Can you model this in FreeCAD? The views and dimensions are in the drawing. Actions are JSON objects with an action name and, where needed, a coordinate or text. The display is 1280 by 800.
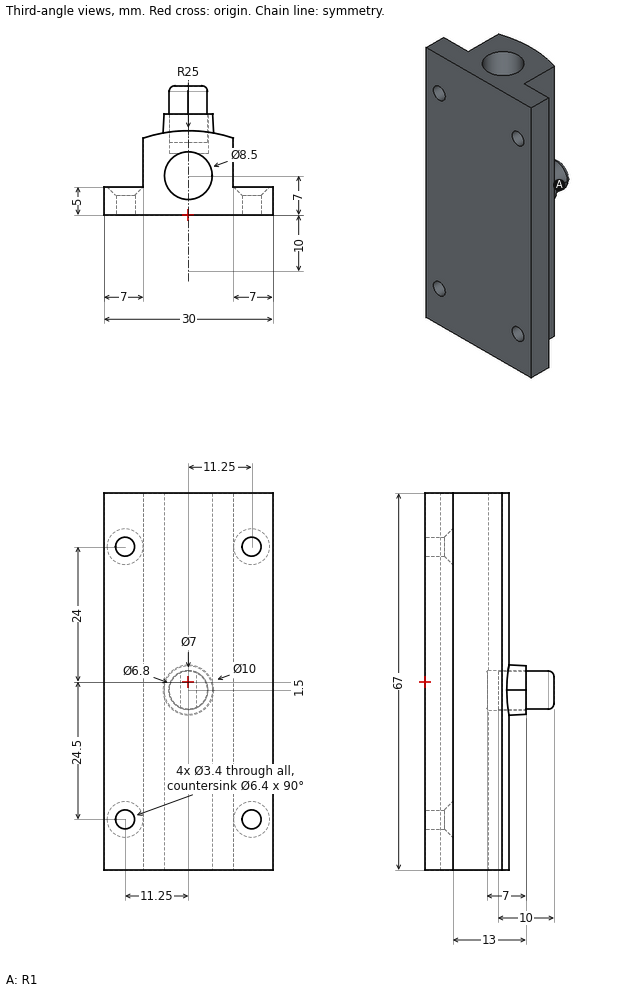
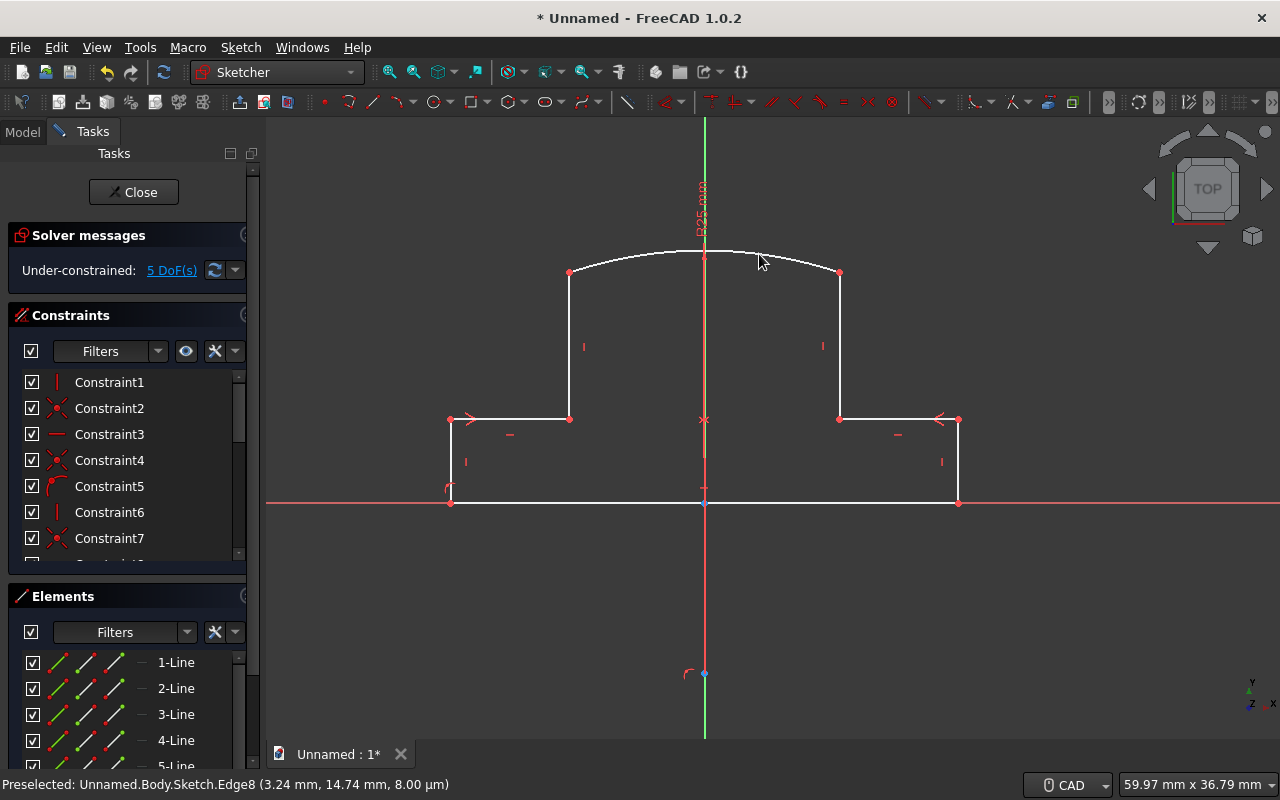
{"action": "left_click", "coordinate": [534, 419]}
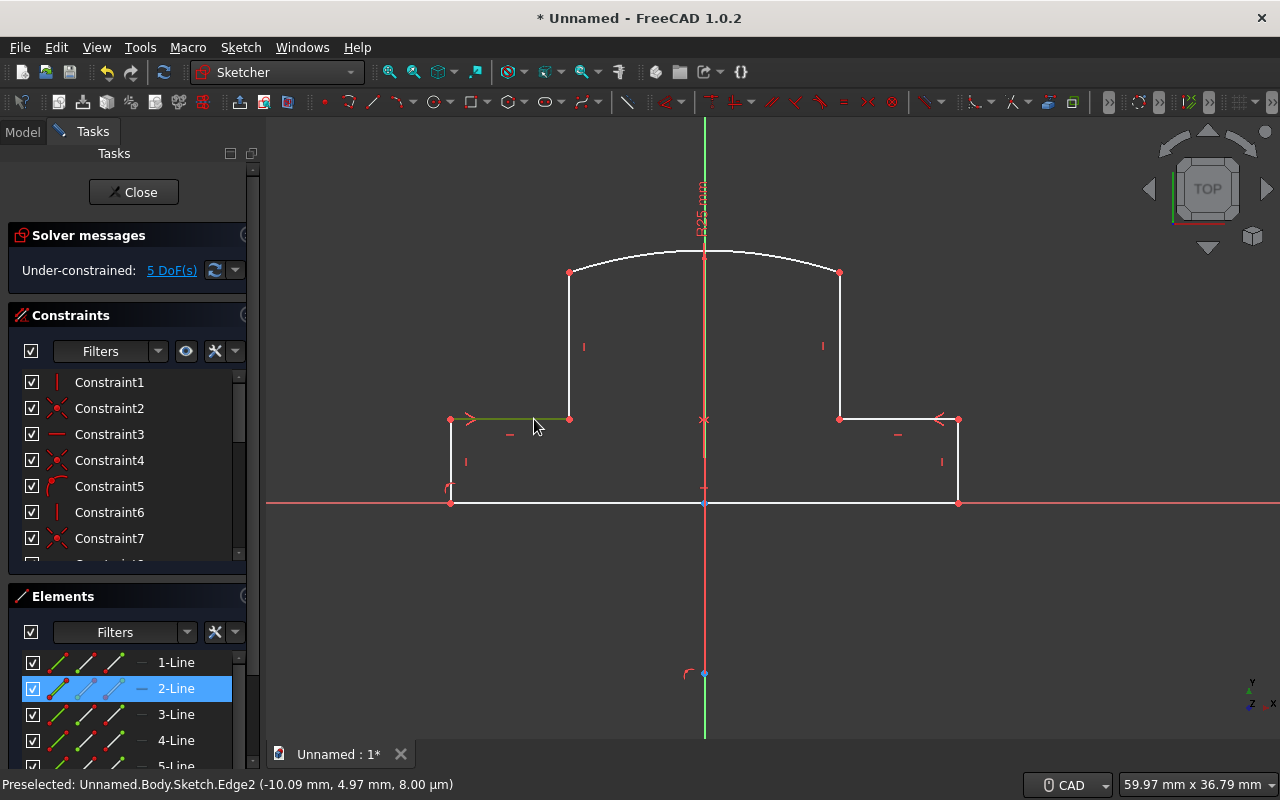
{"action": "left_click", "coordinate": [684, 102]}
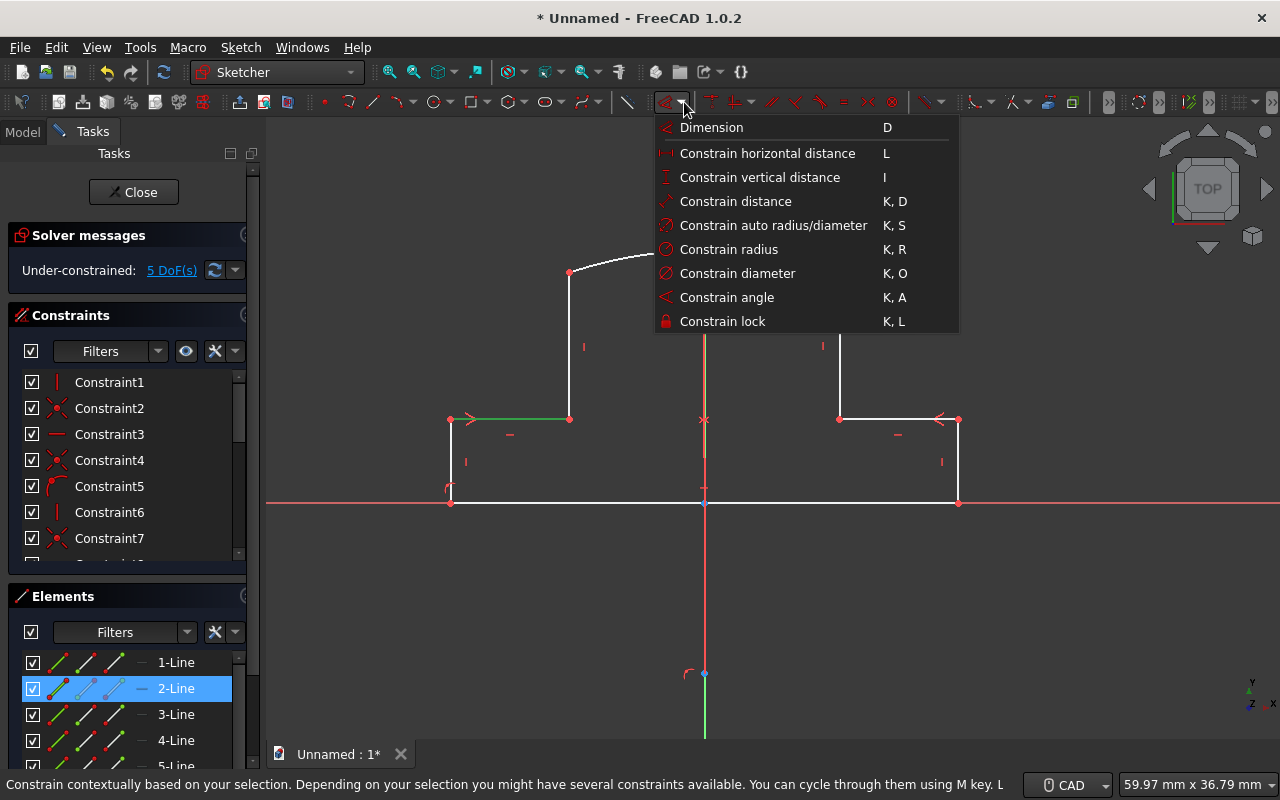
{"action": "left_click", "coordinate": [807, 153]}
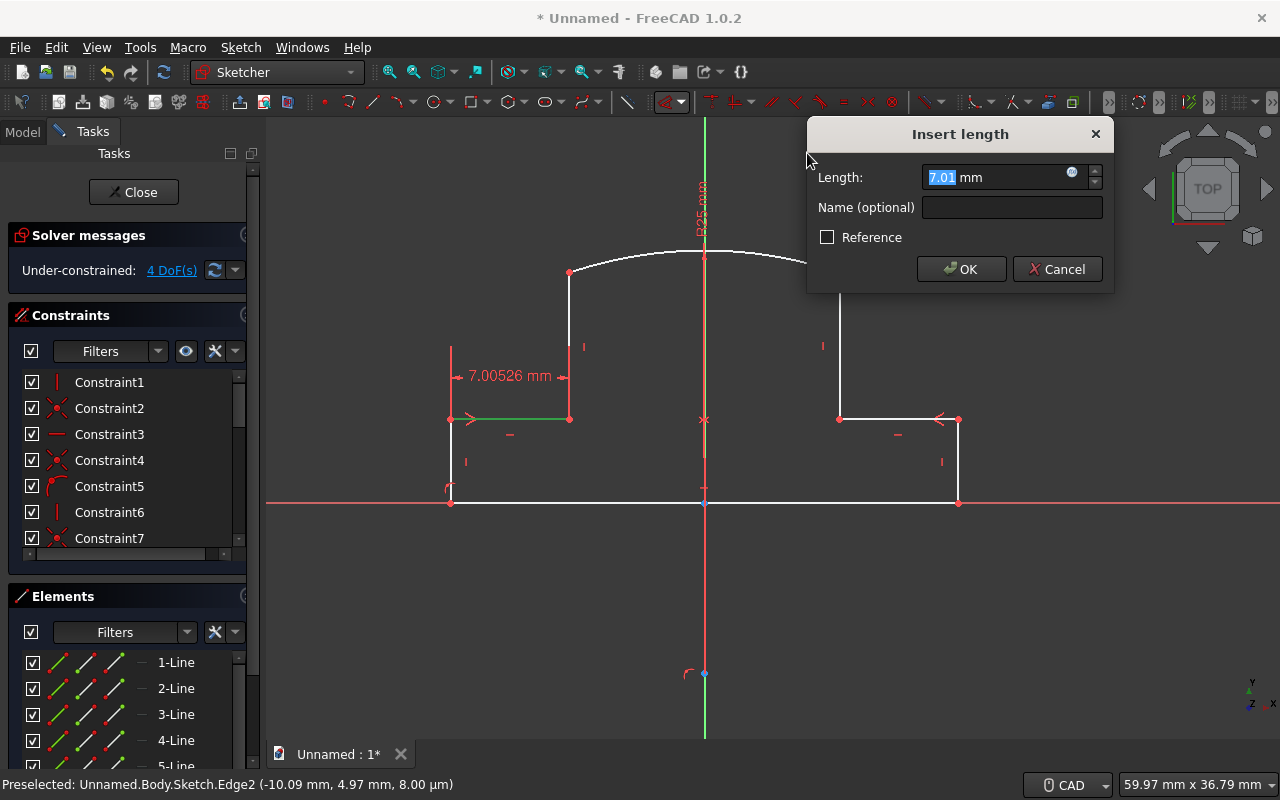
{"action": "type", "text": "7"}
{"action": "key", "text": "Return"}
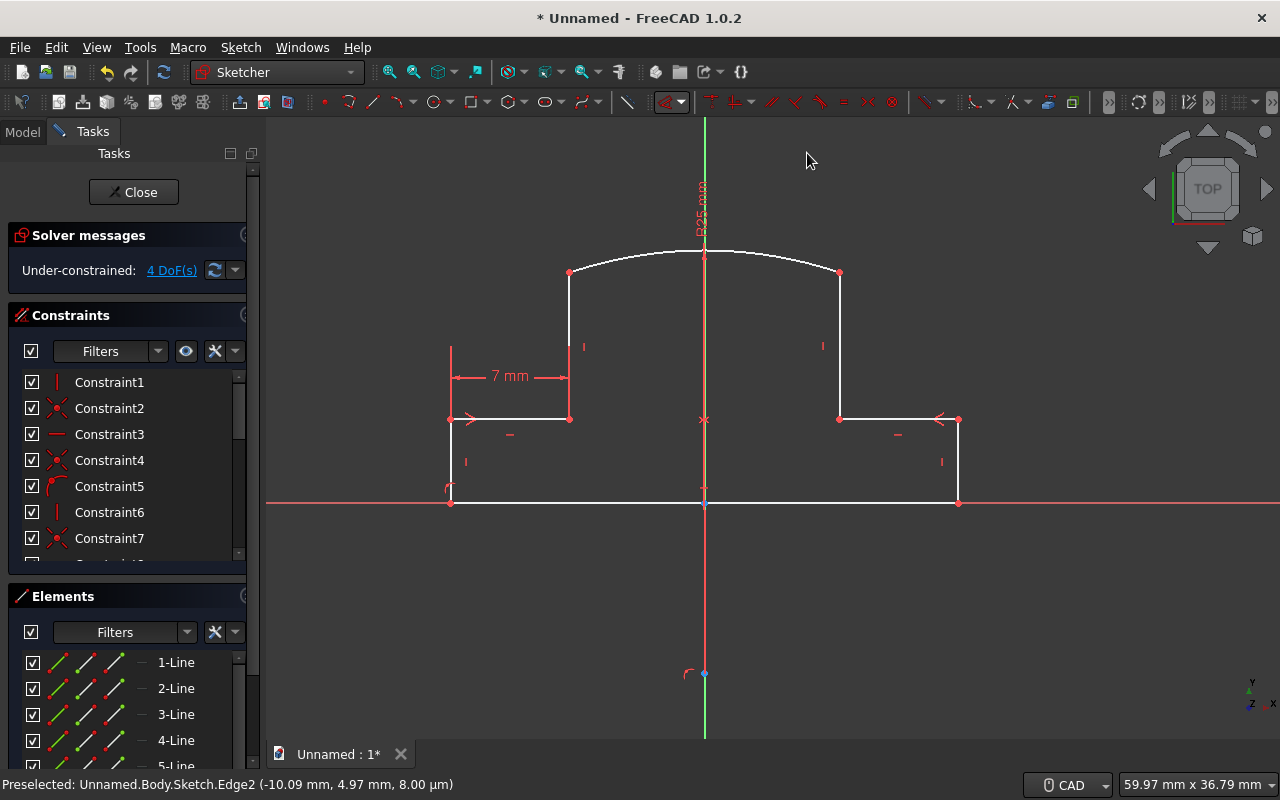
{"action": "left_click", "coordinate": [451, 444]}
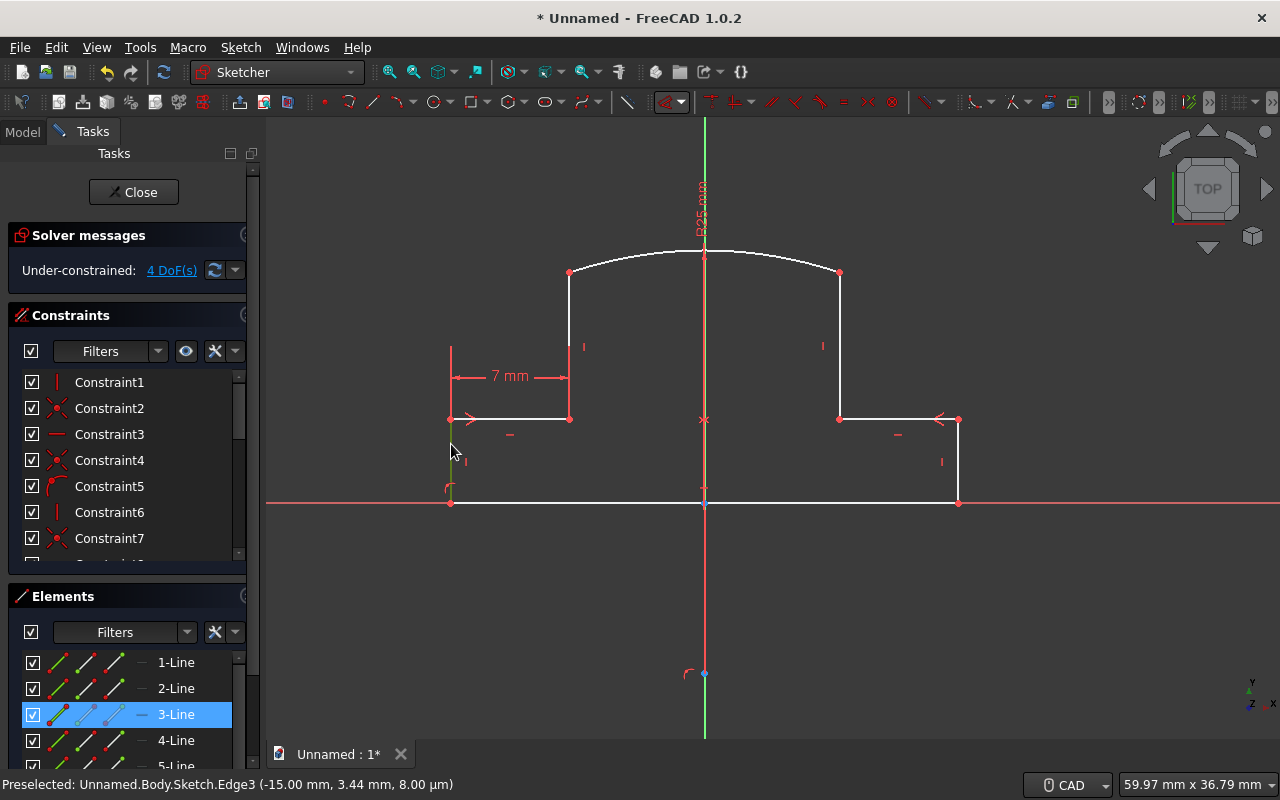
{"action": "key", "text": "i"}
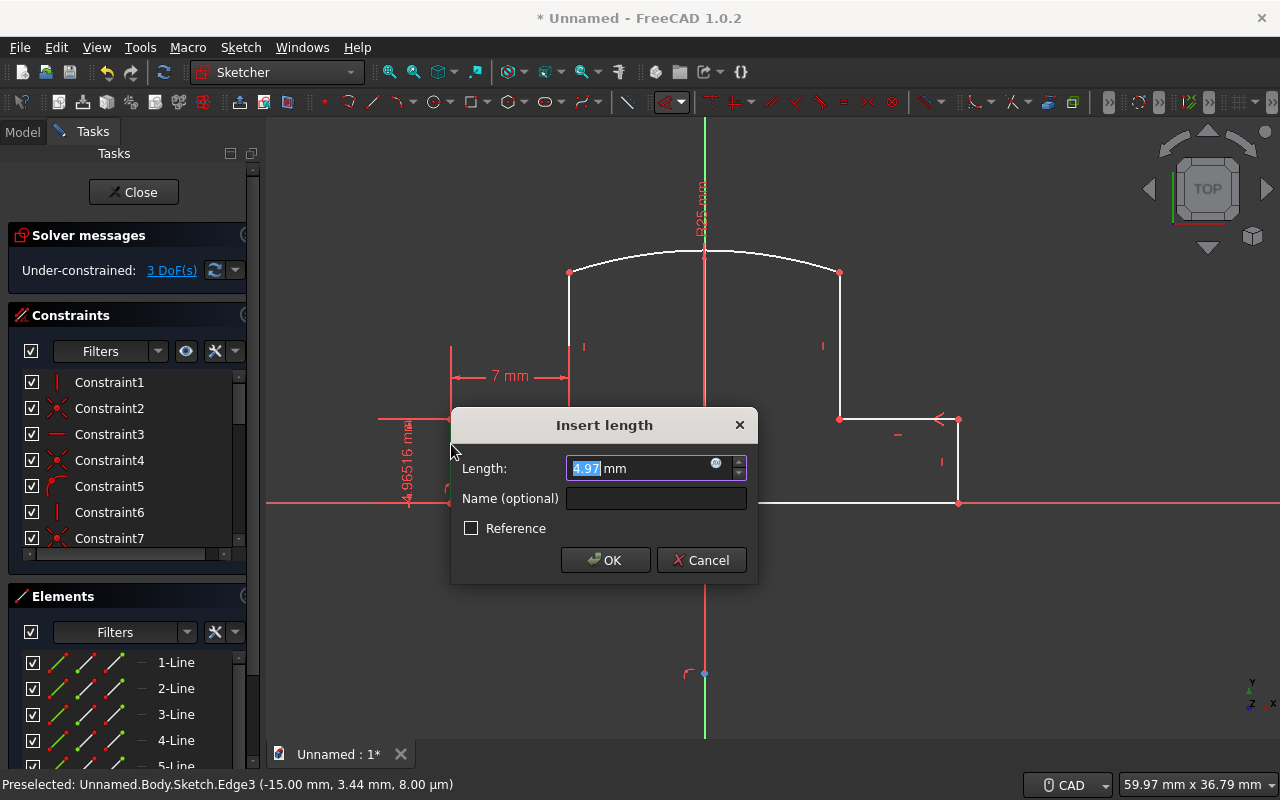
{"action": "type", "text": "5"}
{"action": "key", "text": "Return"}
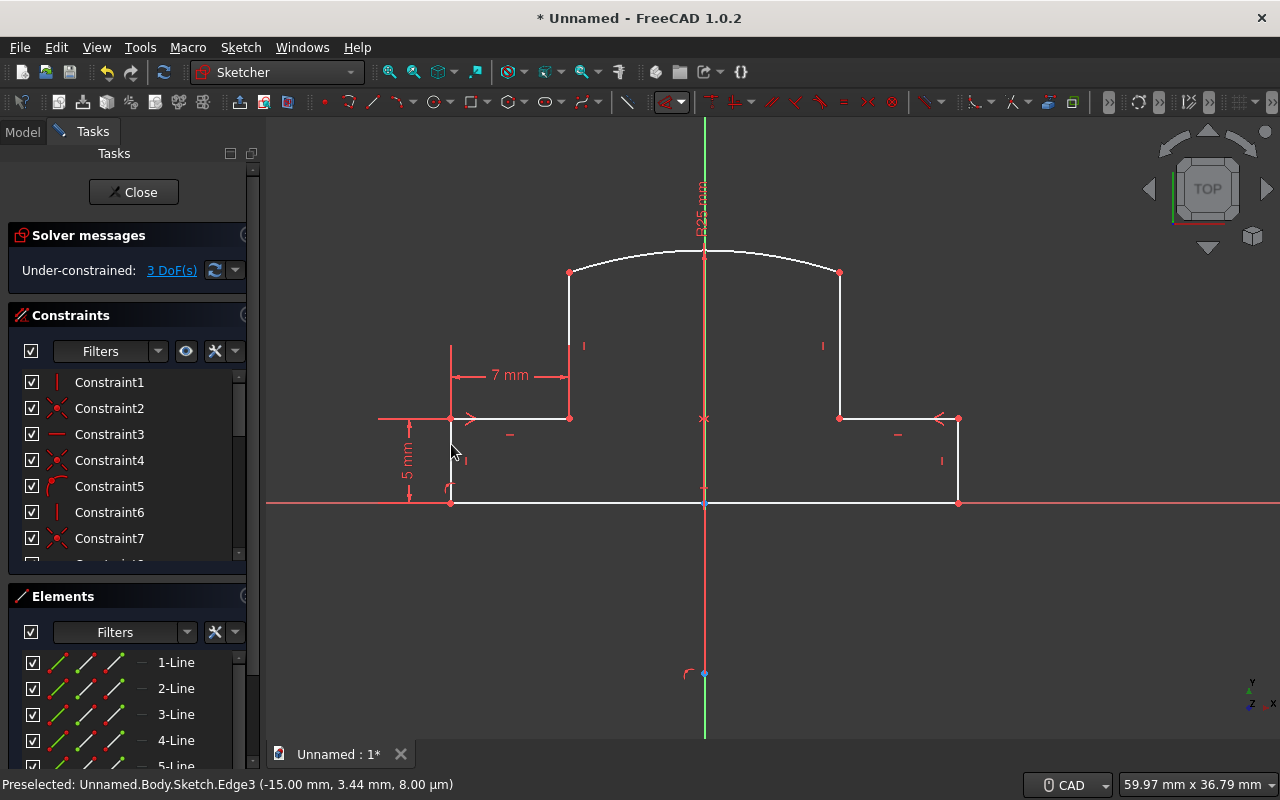
{"action": "left_click", "coordinate": [923, 419]}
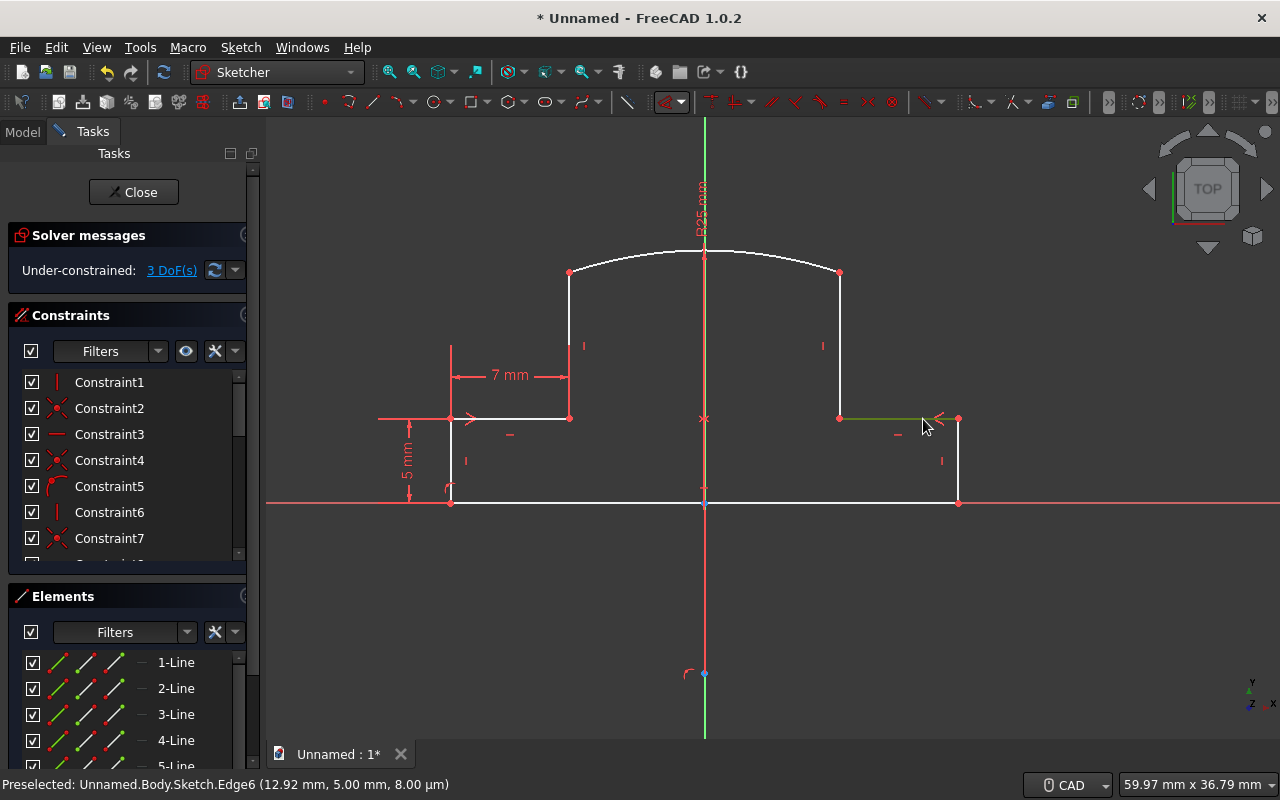
{"action": "key", "text": "l"}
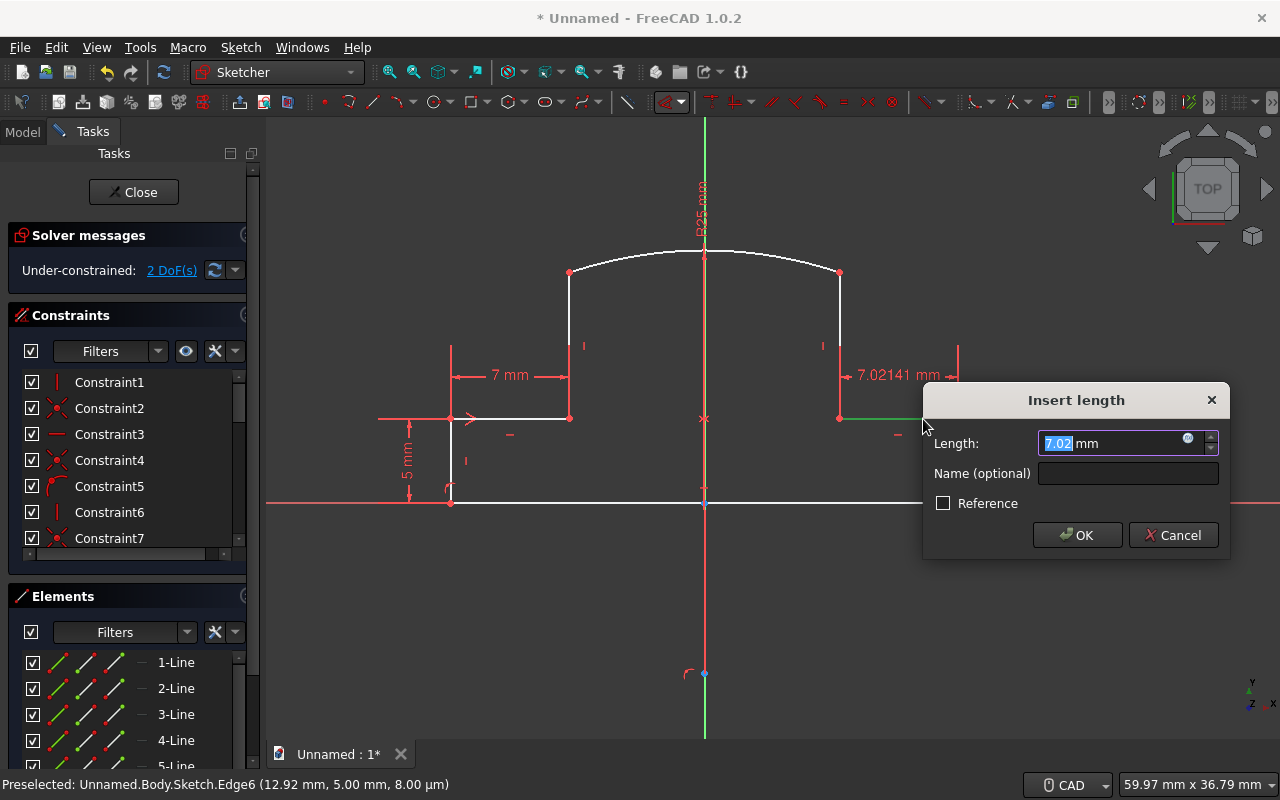
{"action": "type", "text": "7"}
{"action": "key", "text": "Return"}